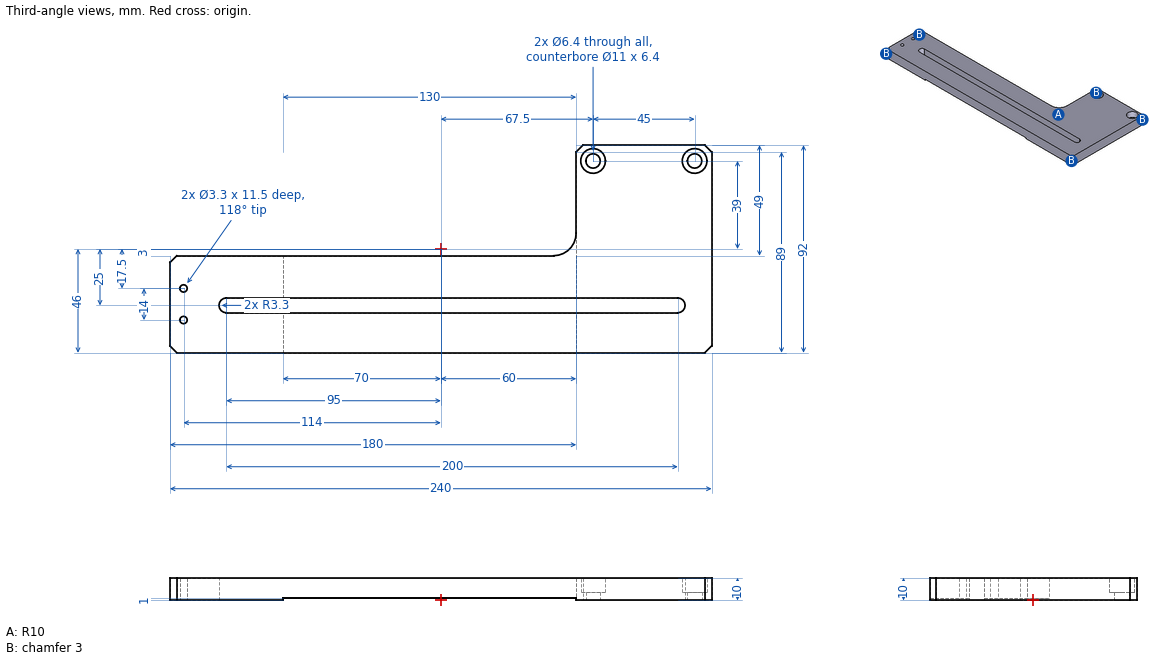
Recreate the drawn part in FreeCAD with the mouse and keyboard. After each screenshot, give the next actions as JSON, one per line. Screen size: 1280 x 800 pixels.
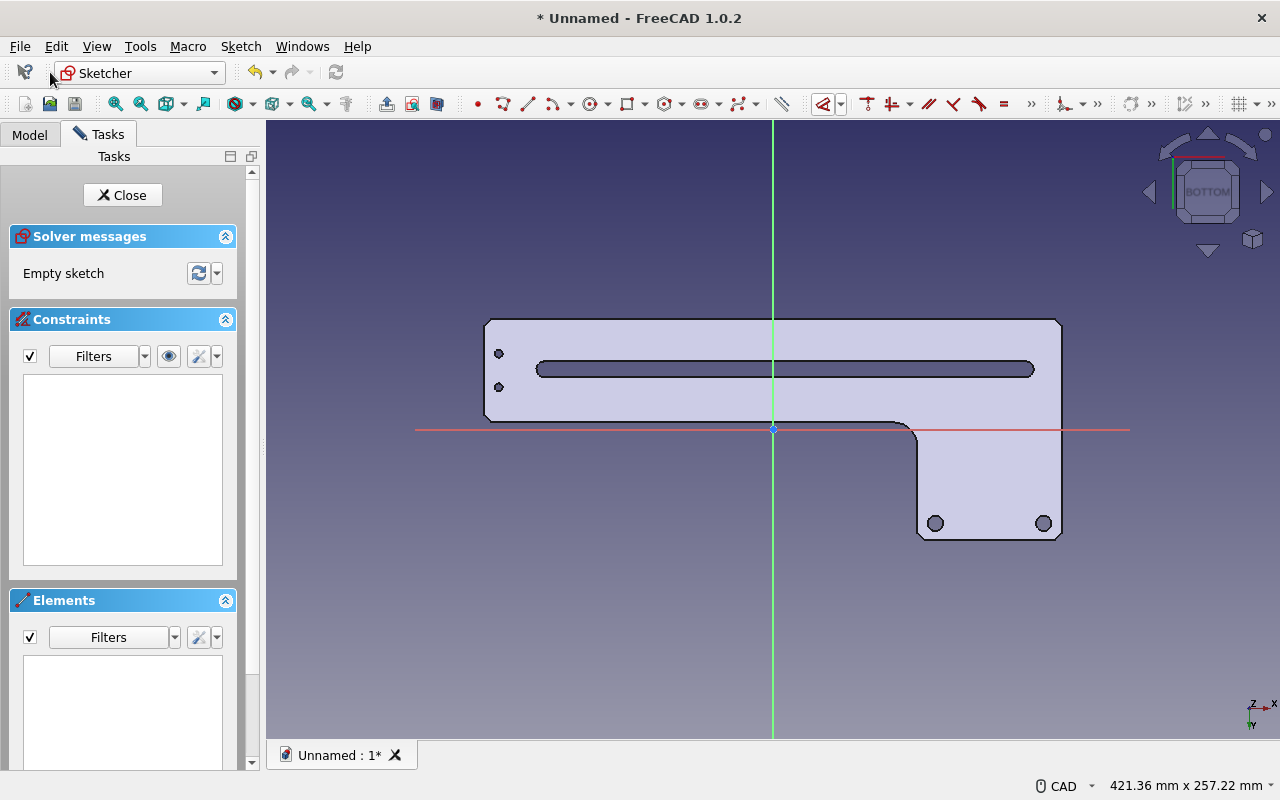
{"action": "scroll", "coordinate": [830, 421], "scroll_direction": "up", "scroll_amount": 3}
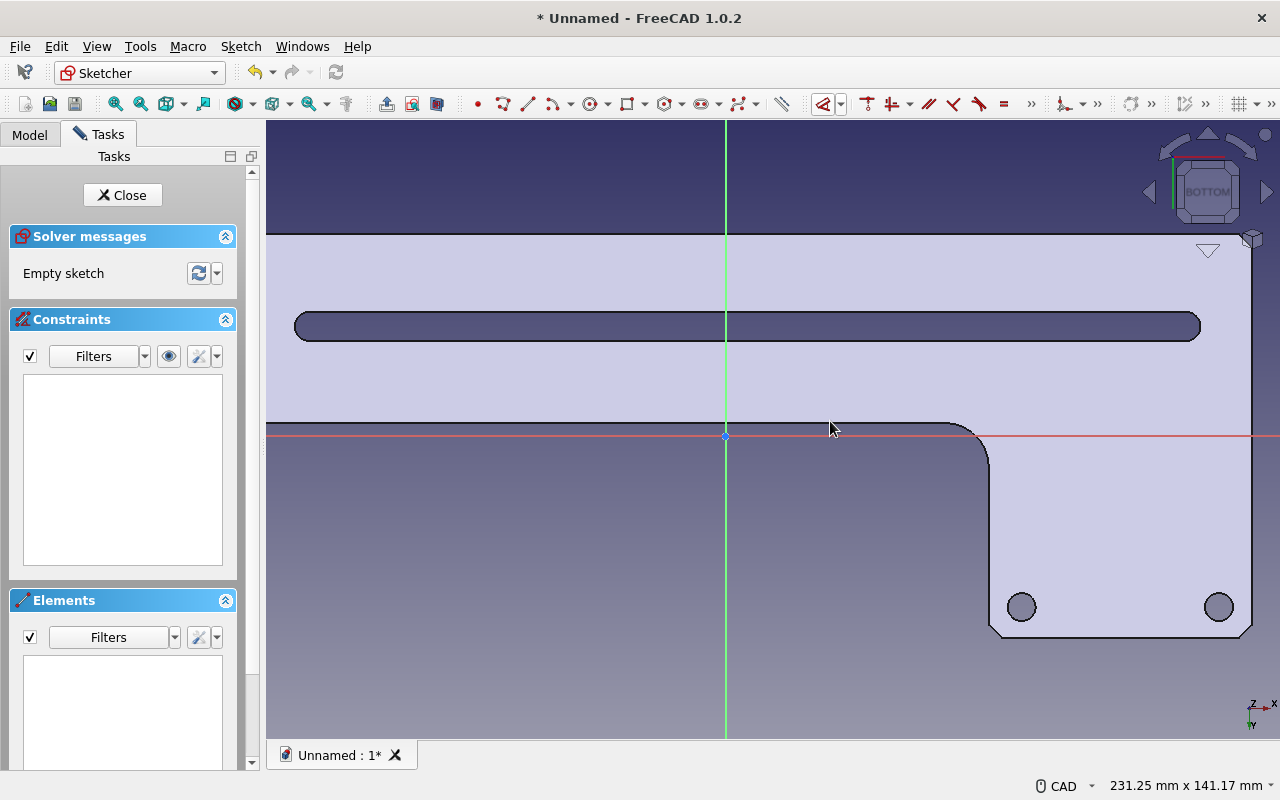
{"action": "key", "text": "g r"}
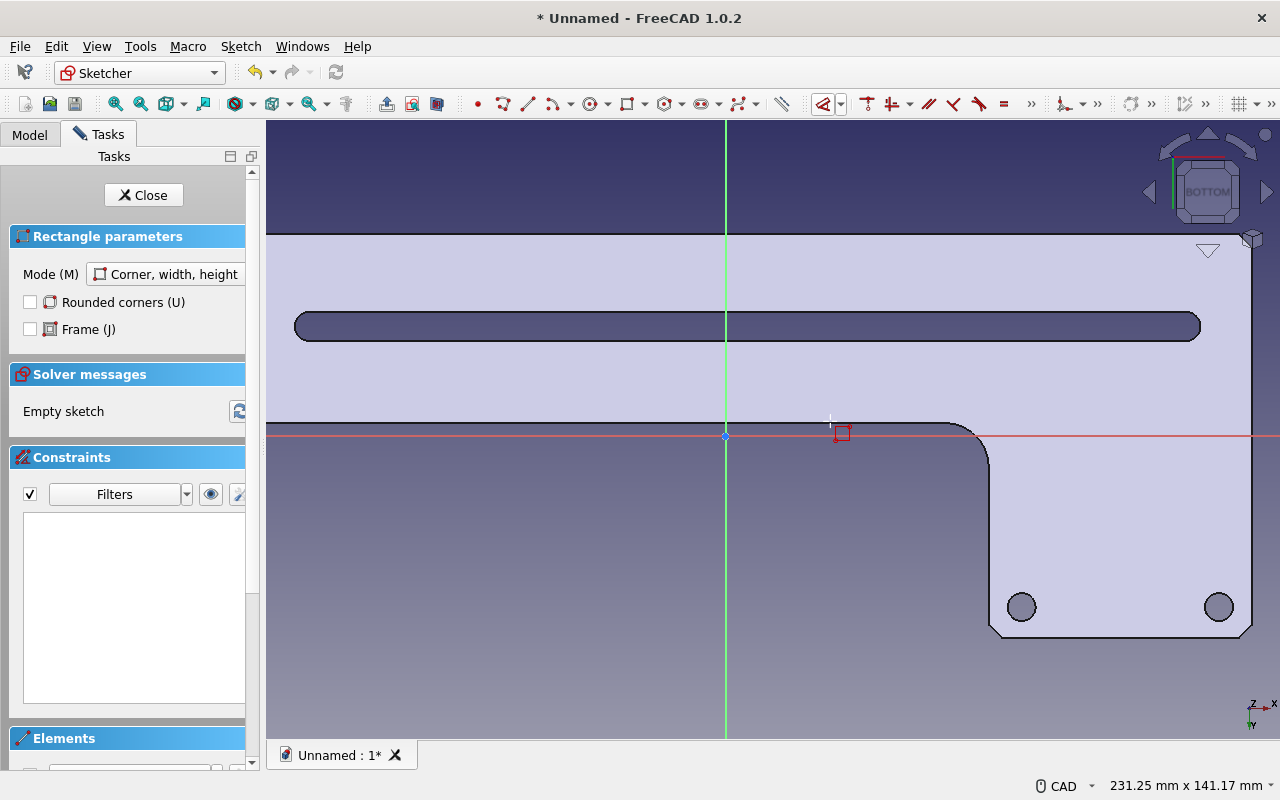
{"action": "left_click", "coordinate": [419, 234]}
{"action": "mouse_move", "coordinate": [989, 625]}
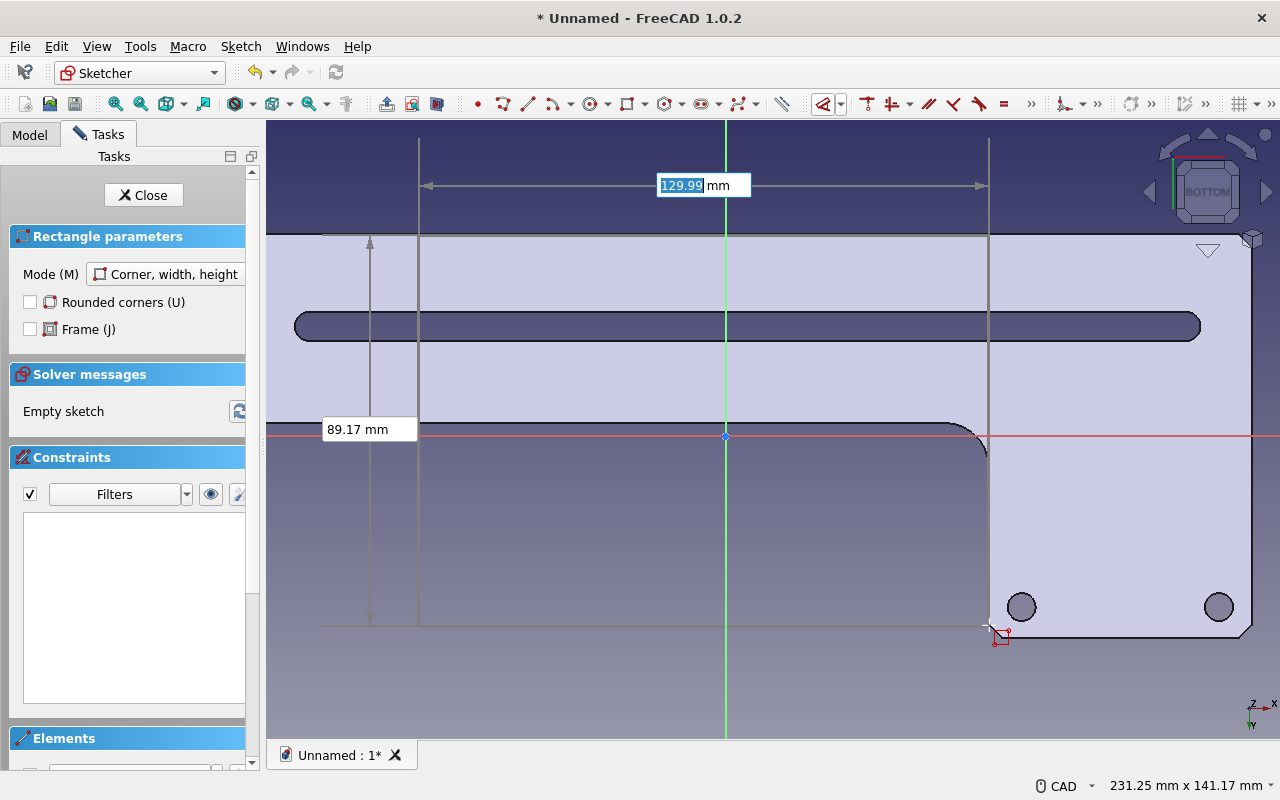
{"action": "type", "text": "130"}
{"action": "key", "text": "Tab"}
{"action": "type", "text": "89"}
{"action": "key", "text": "Return"}
{"action": "key", "text": "Escape"}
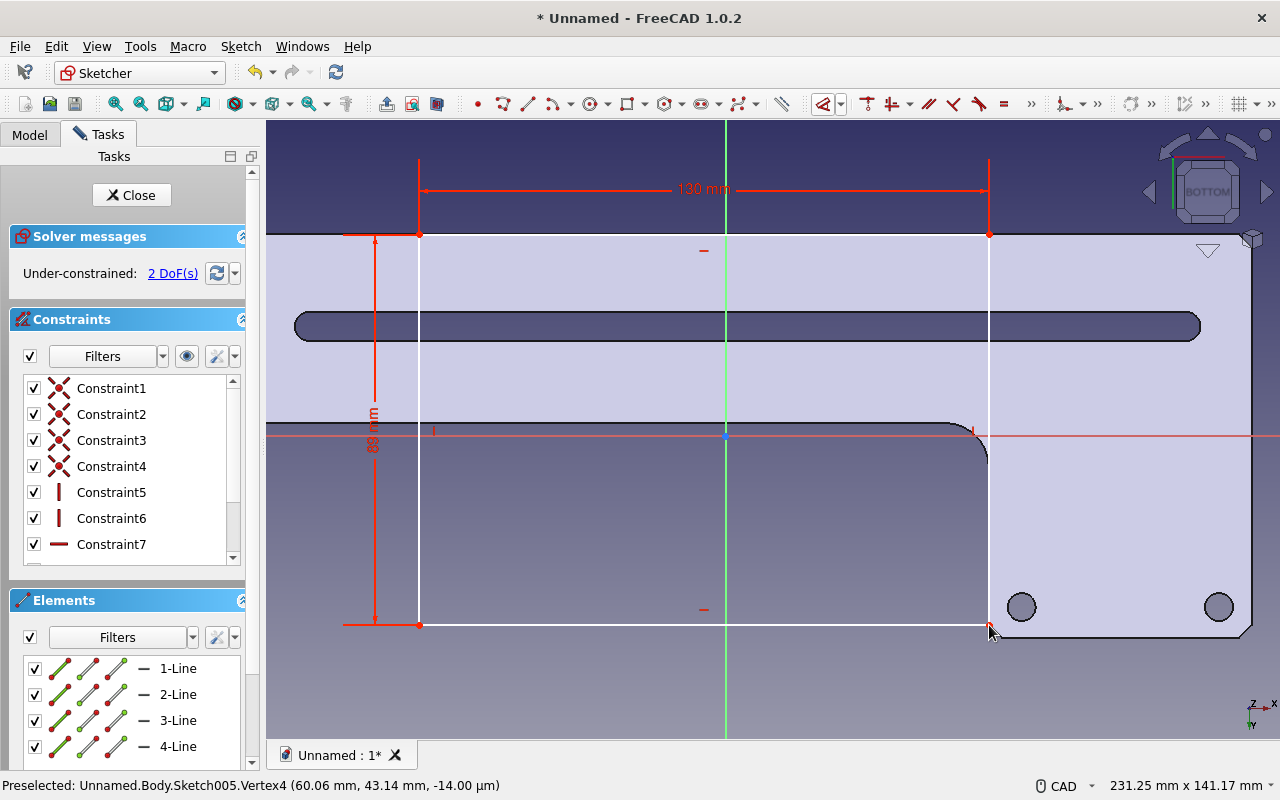
{"action": "left_click", "coordinate": [419, 235]}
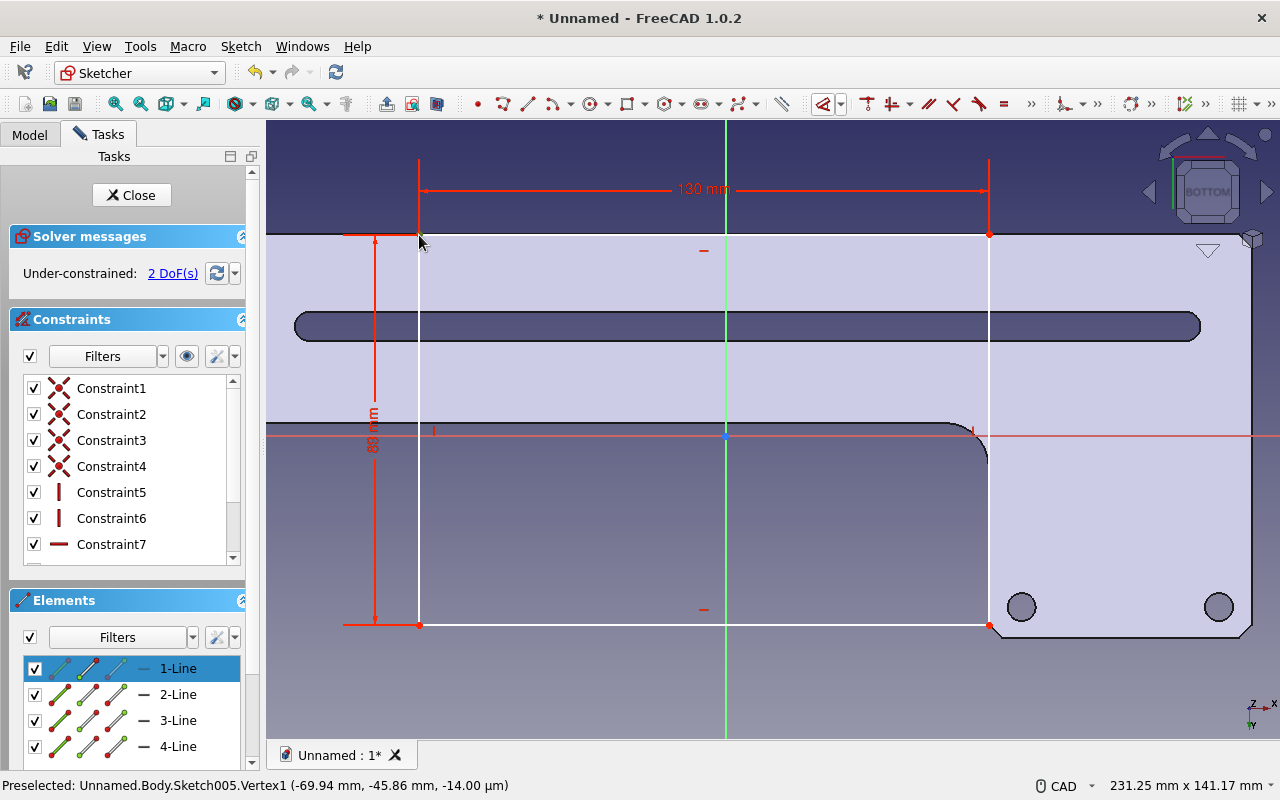
{"action": "key", "text": "l"}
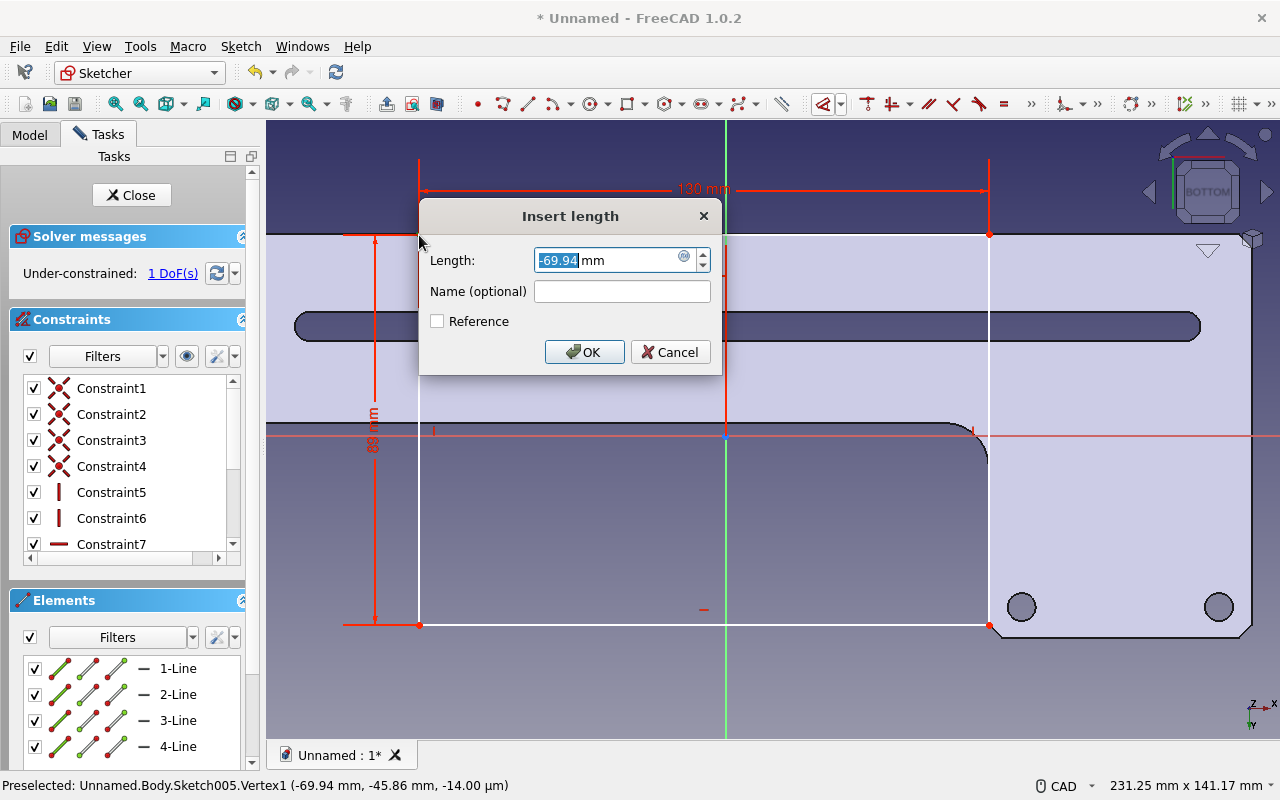
{"action": "type", "text": "-70"}
{"action": "key", "text": "Return"}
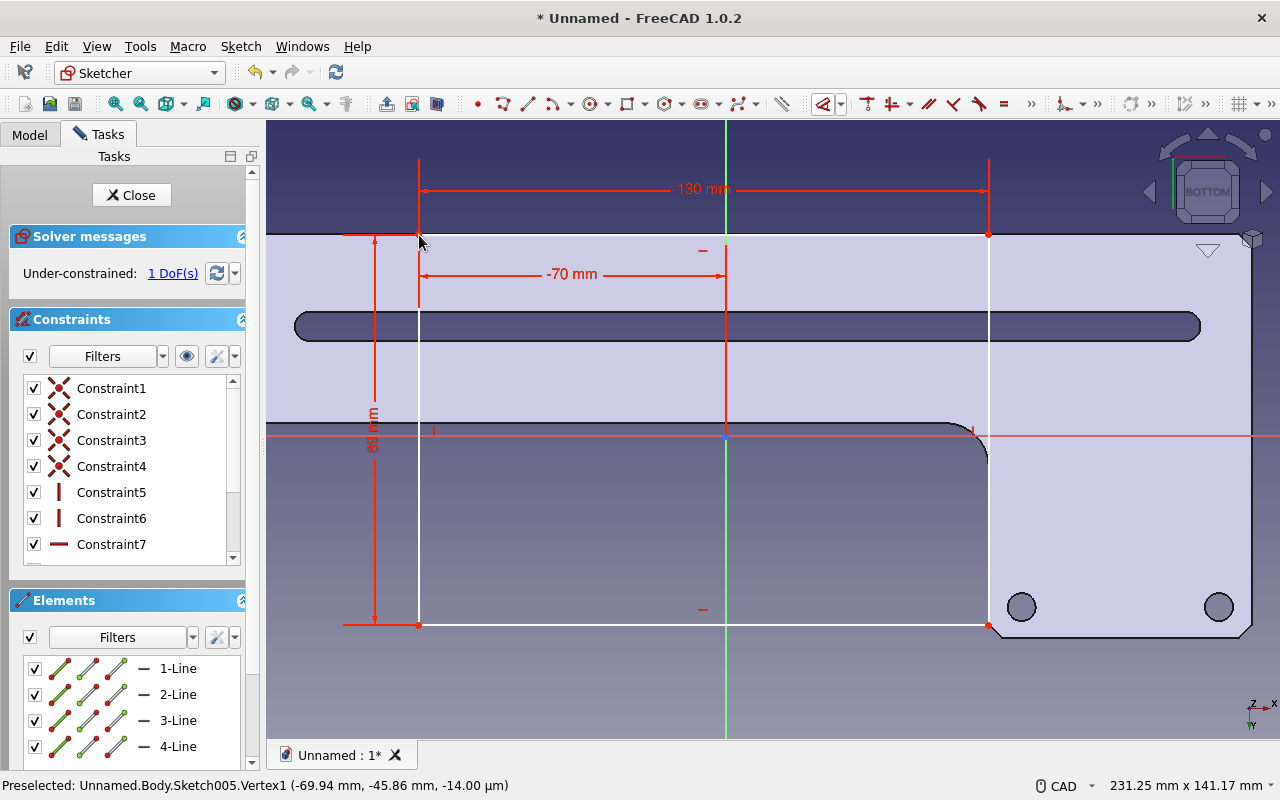
{"action": "left_click", "coordinate": [419, 235]}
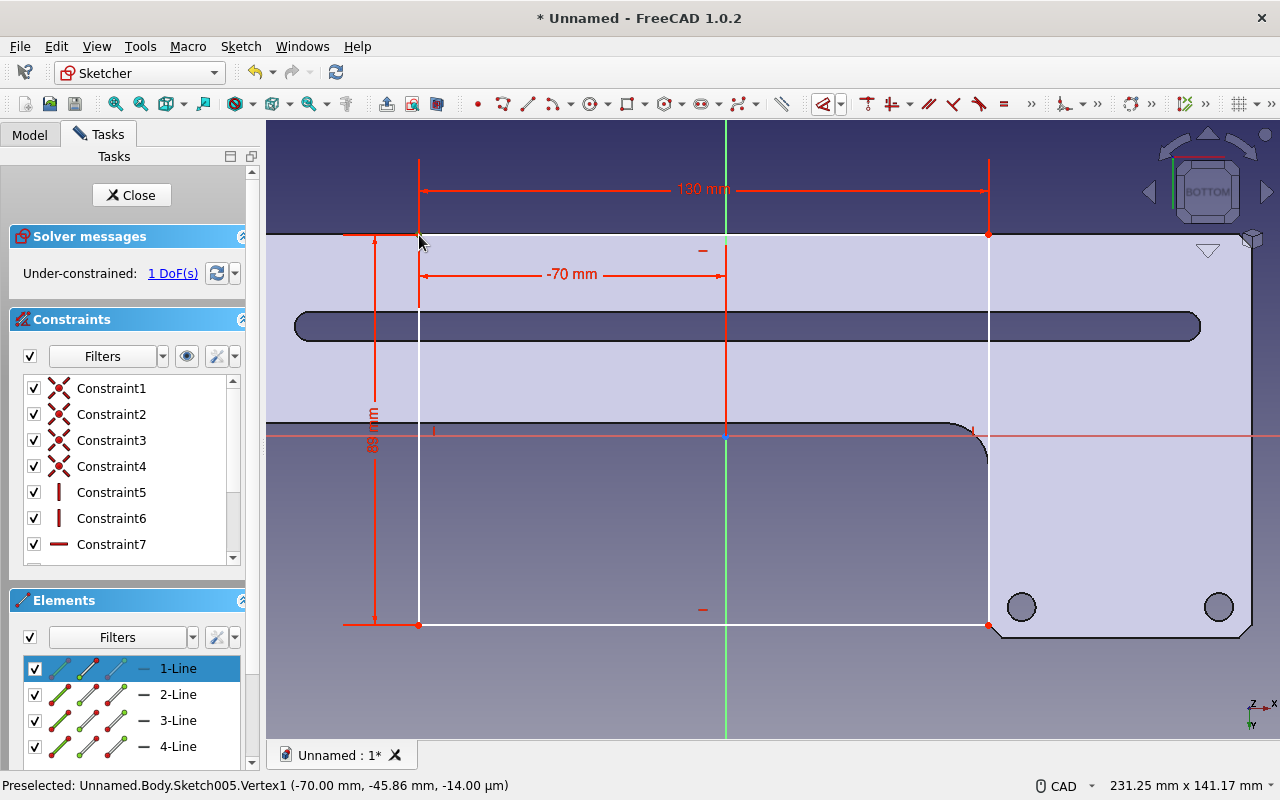
{"action": "key", "text": "i"}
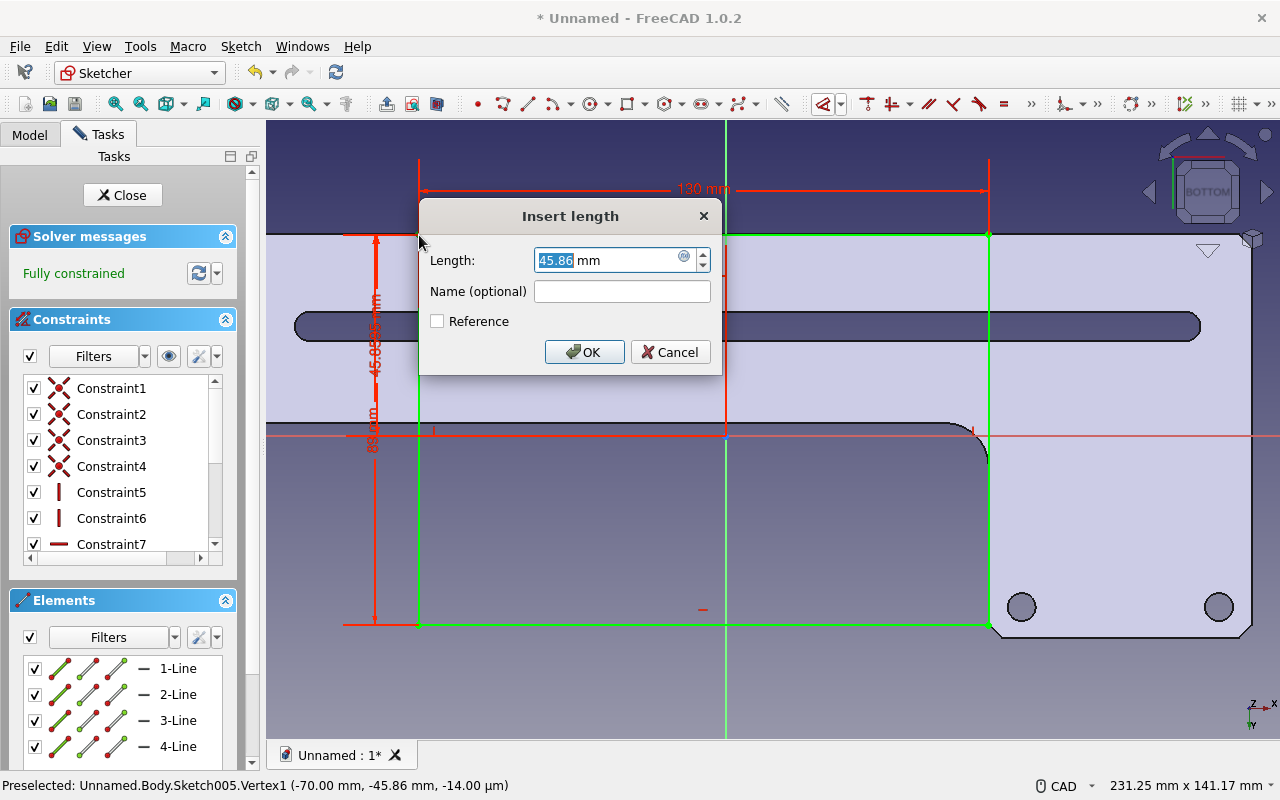
{"action": "type", "text": "46"}
{"action": "key", "text": "Return"}